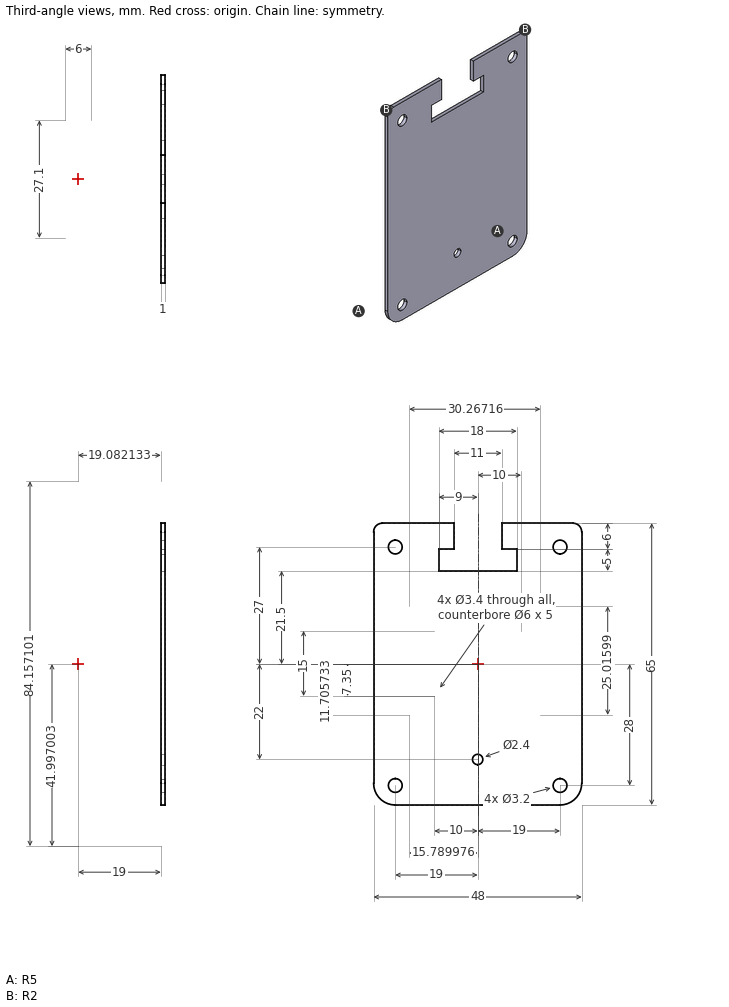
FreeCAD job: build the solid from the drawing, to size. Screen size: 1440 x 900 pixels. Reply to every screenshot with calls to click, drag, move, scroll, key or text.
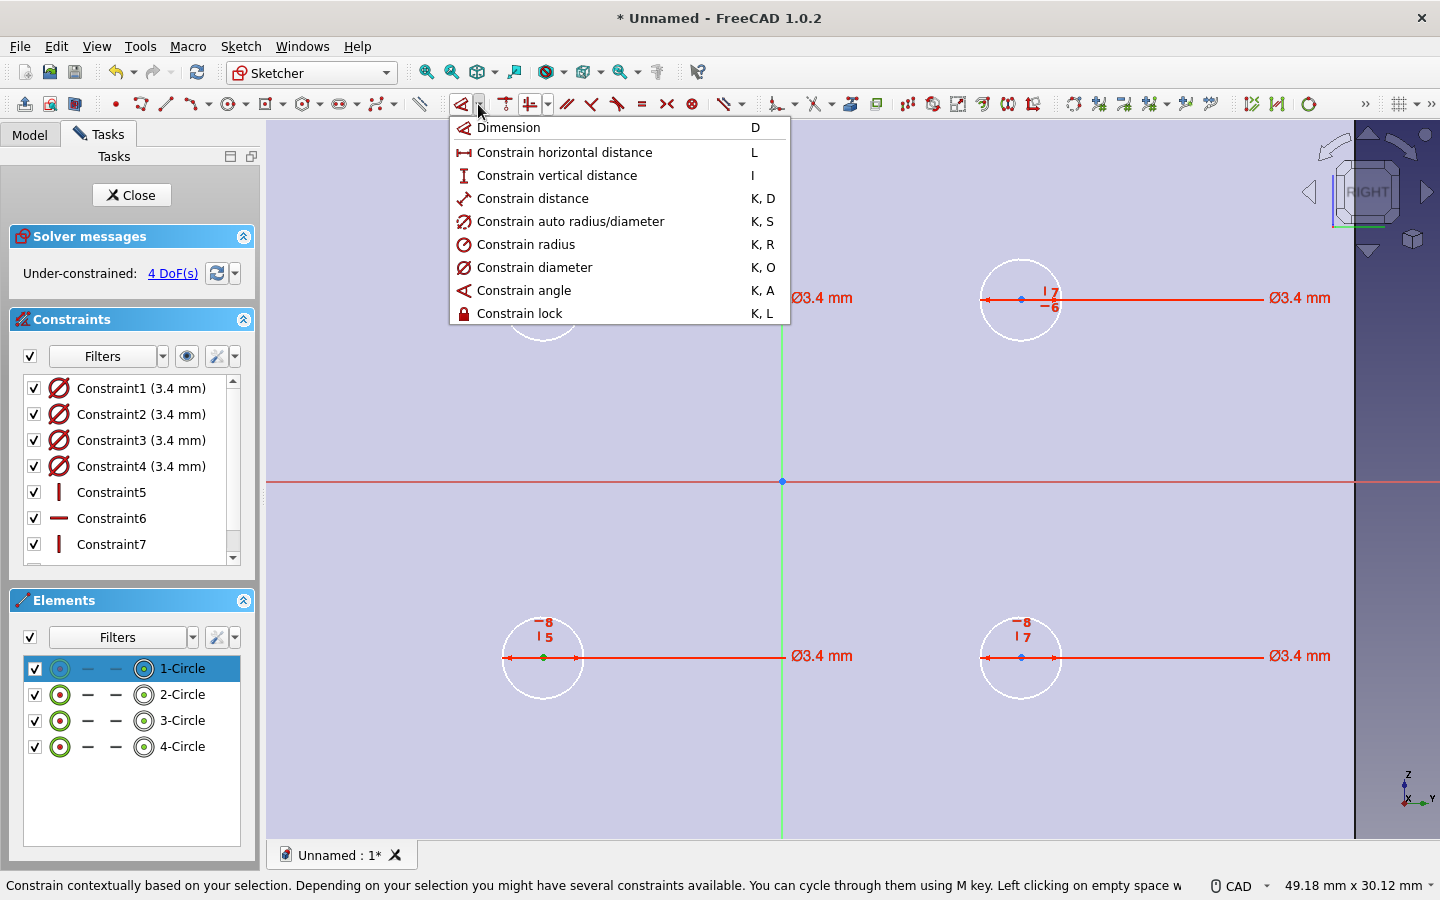
click(620, 152)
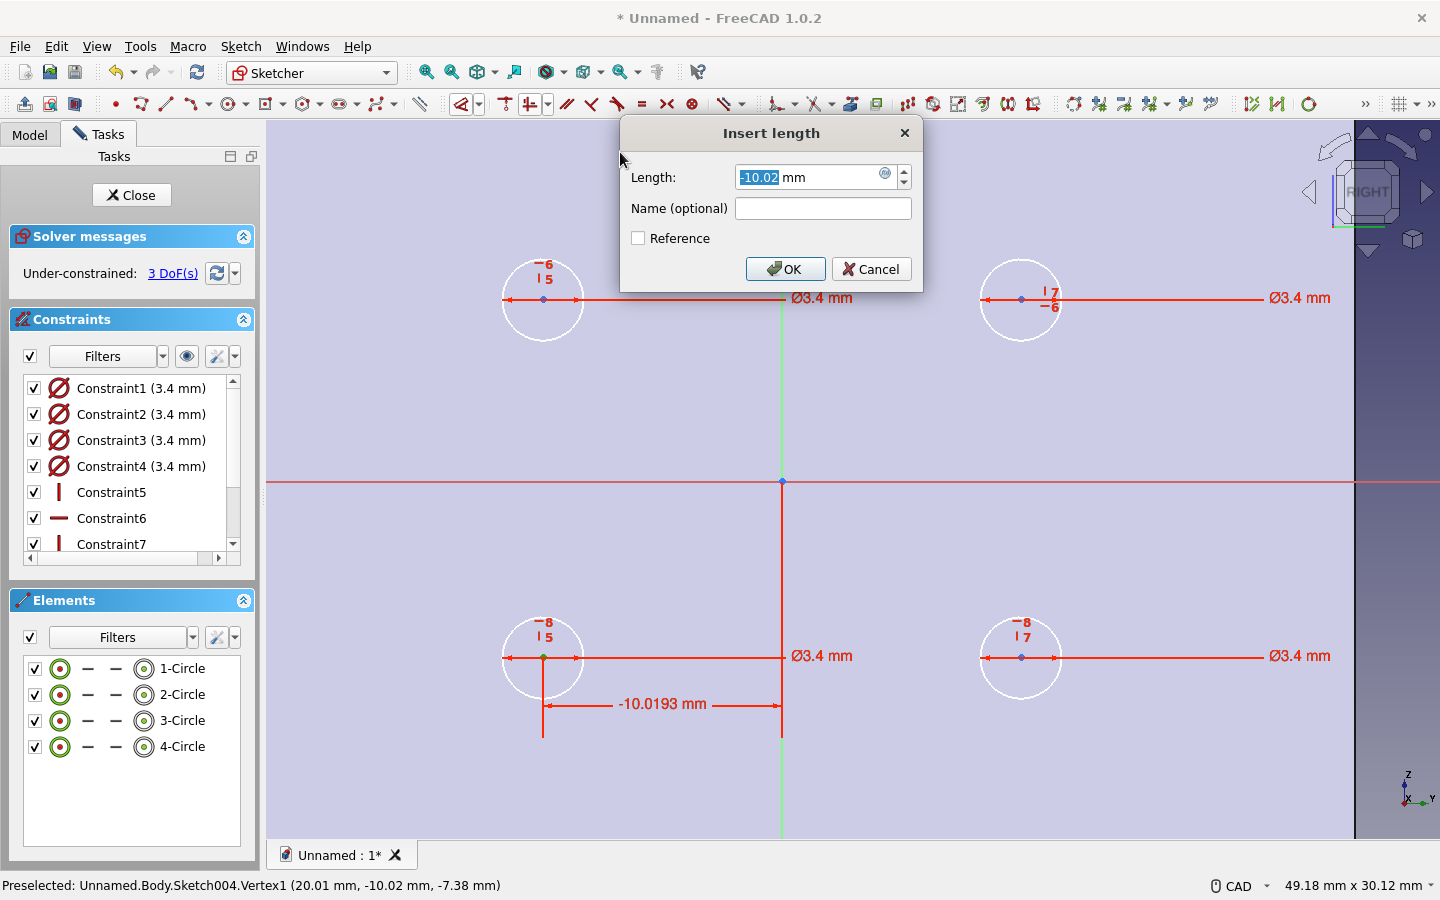
text(-10)
key(Return)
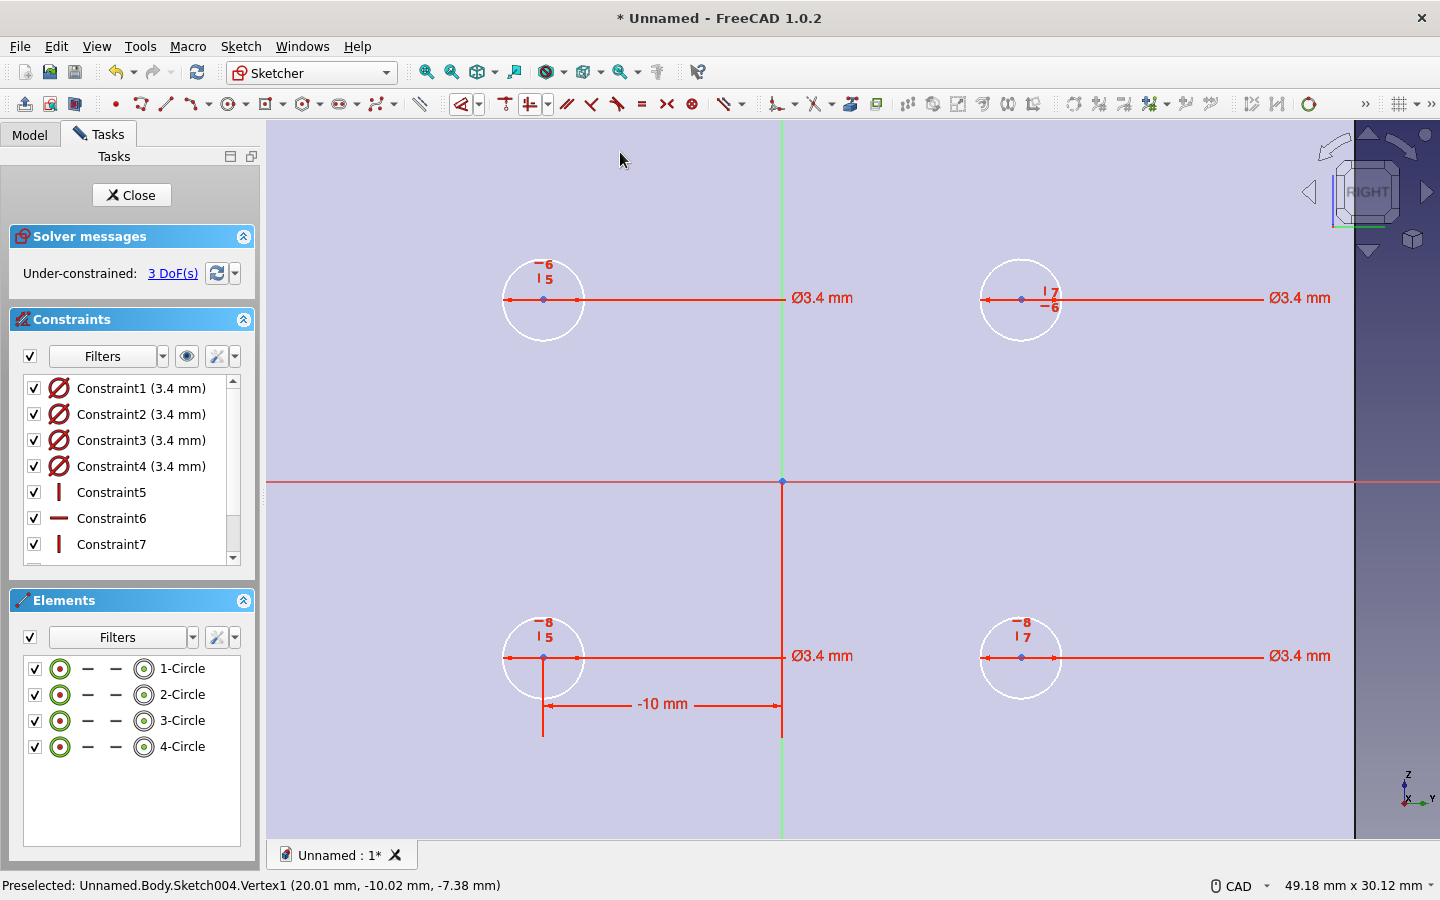
click(1021, 300)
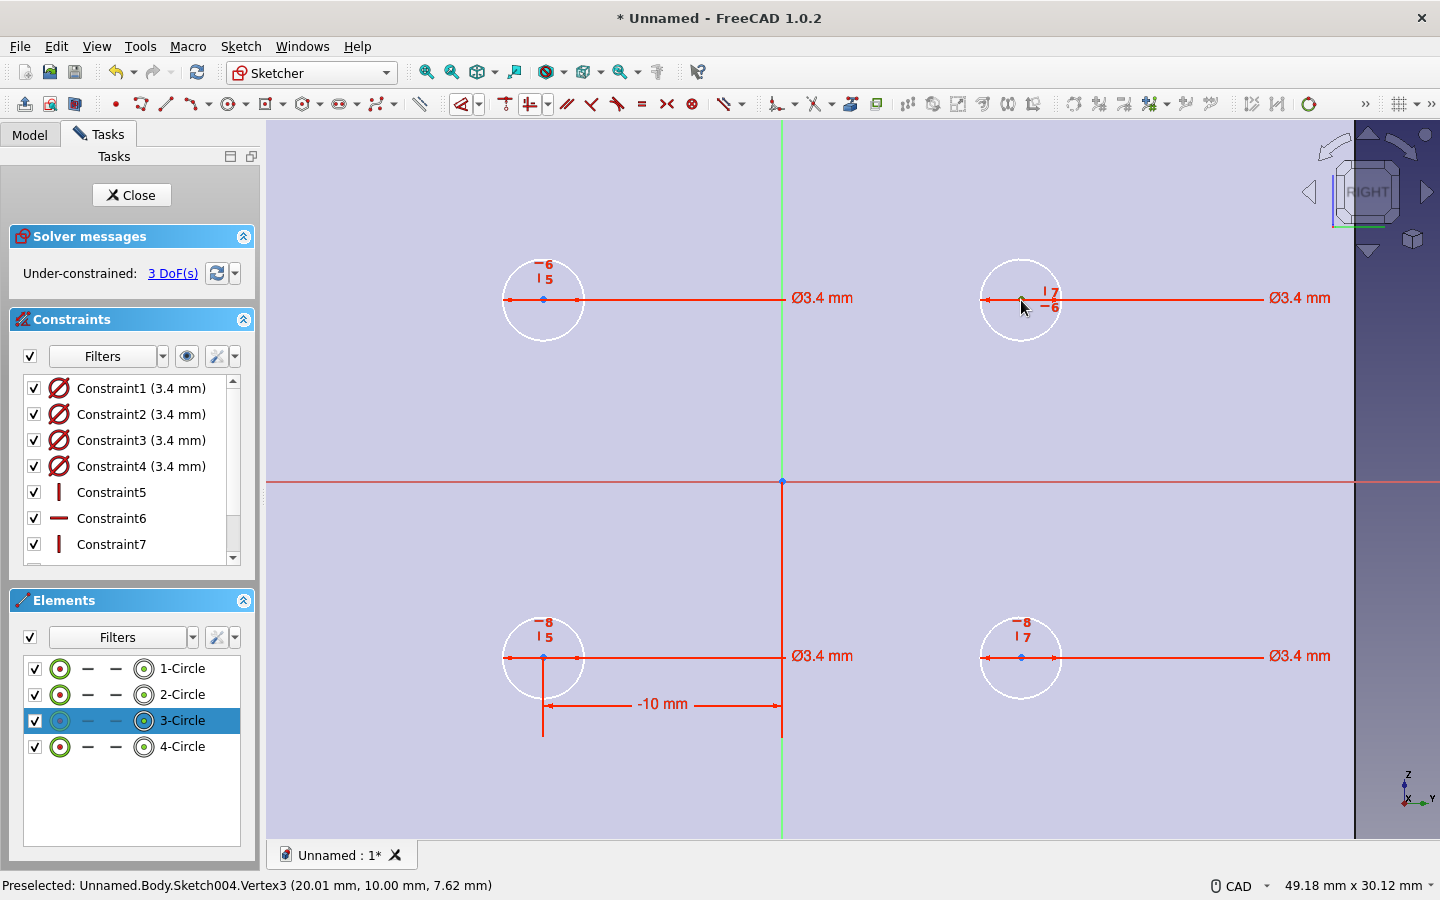
key(l)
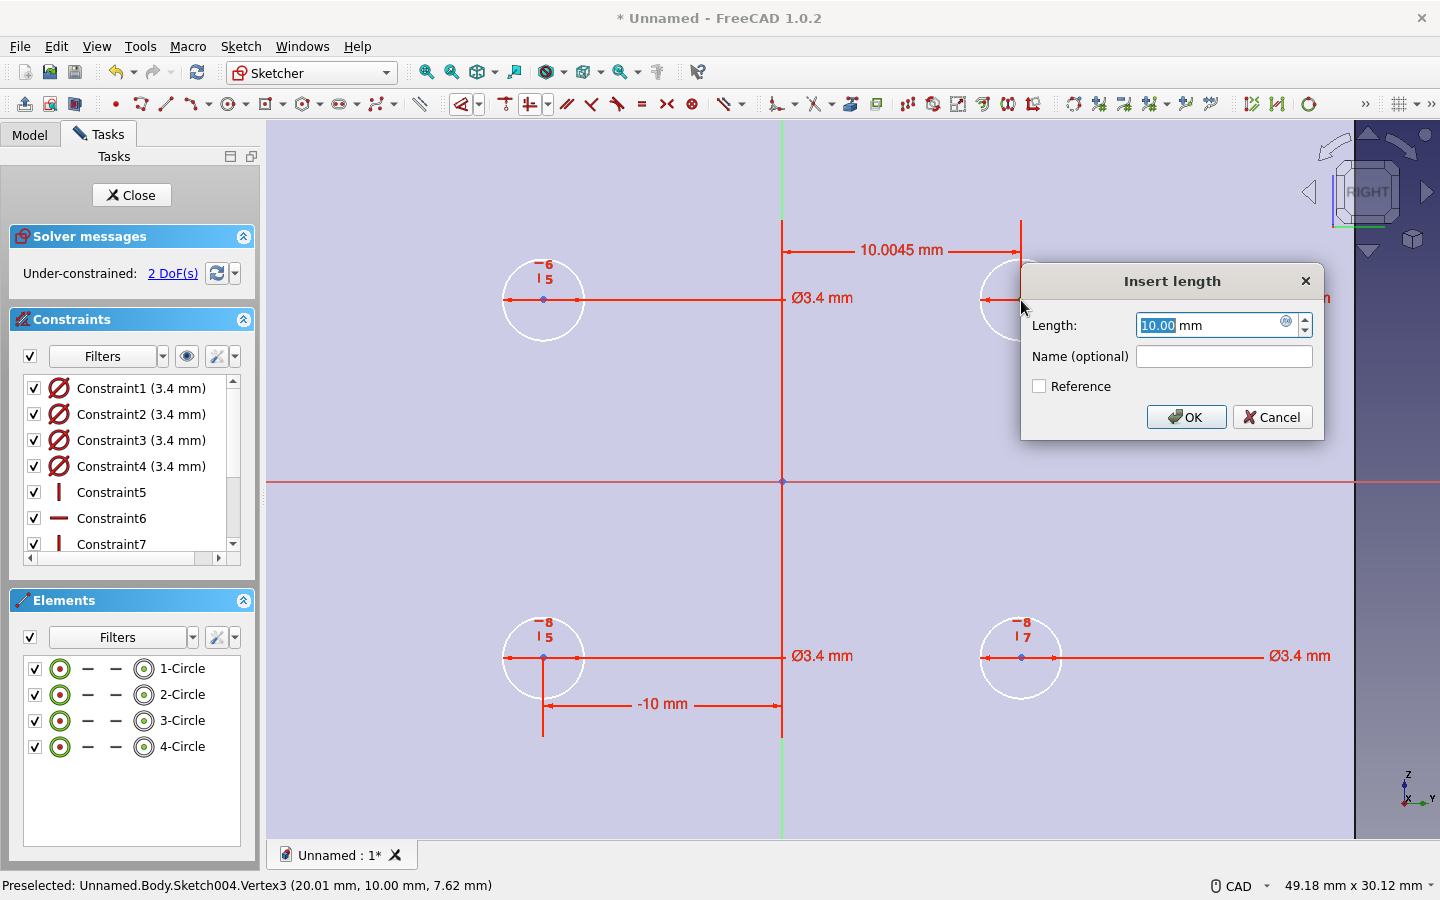
text(10)
key(Return)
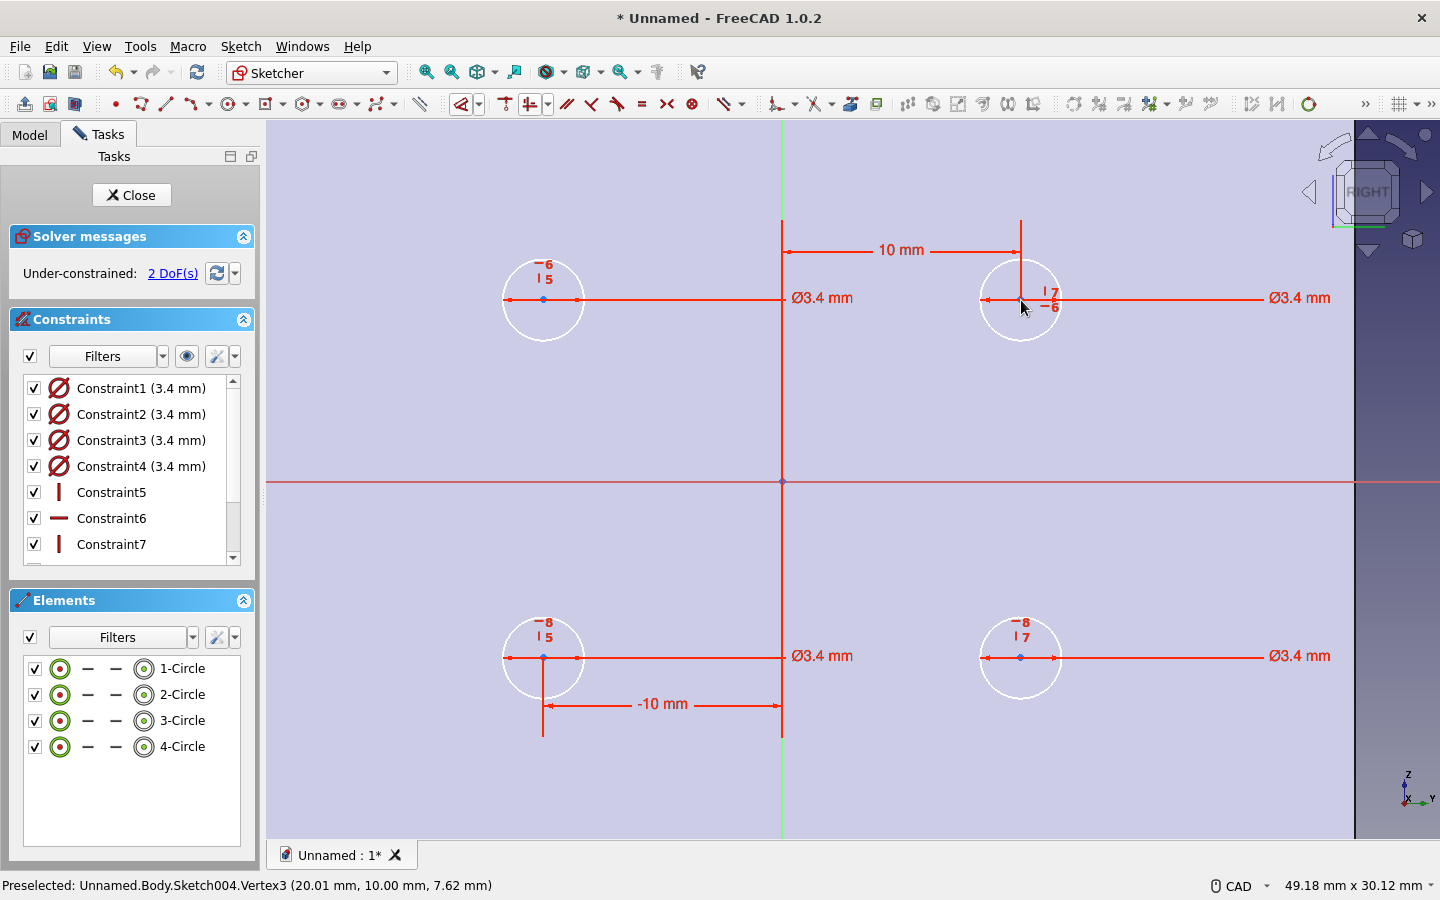
click(543, 658)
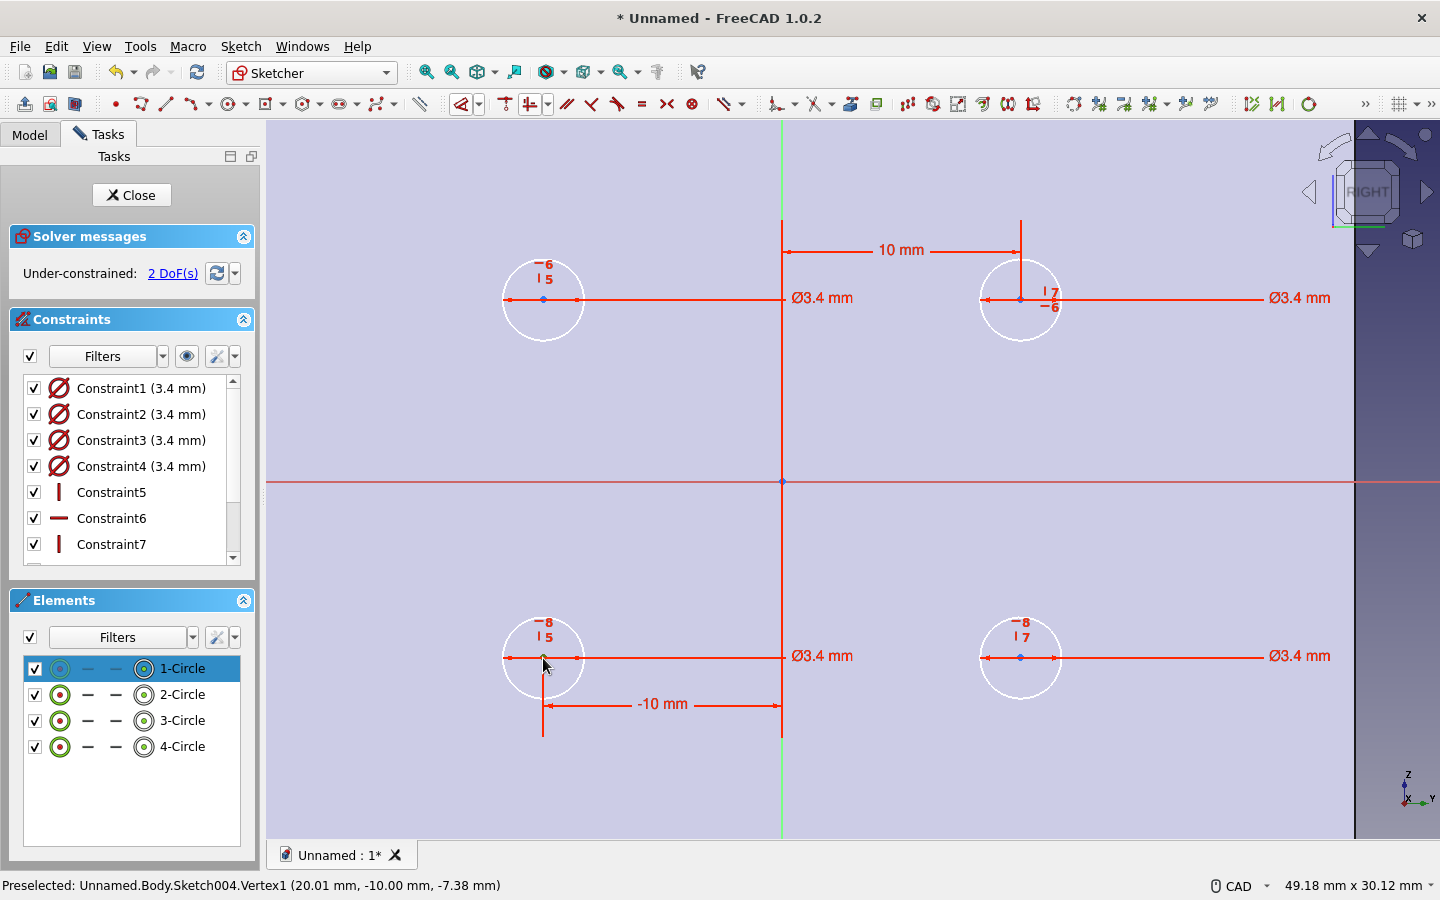
click(543, 300)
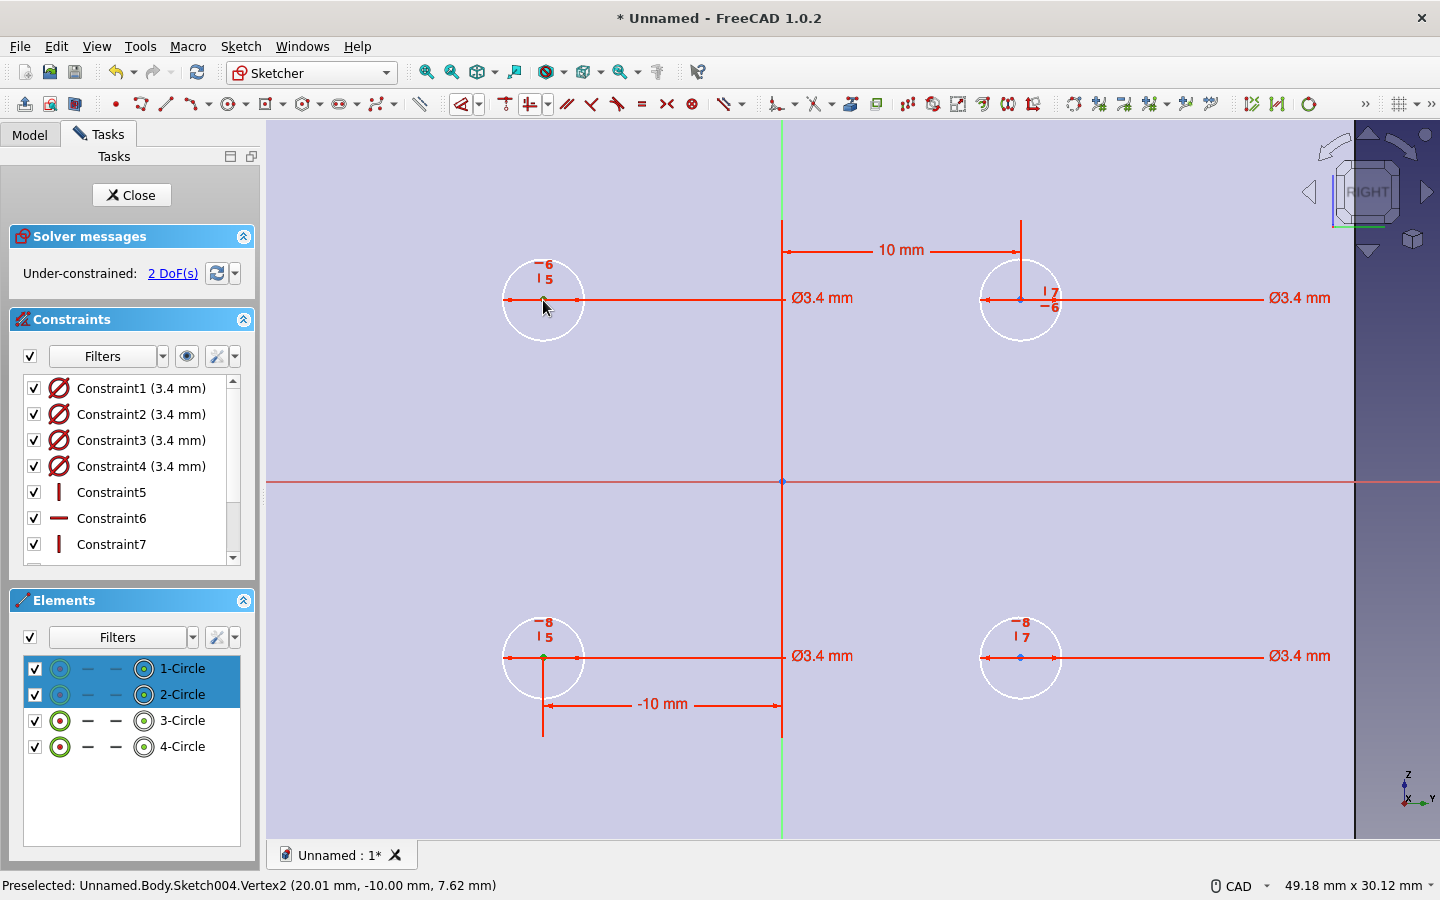
click(478, 104)